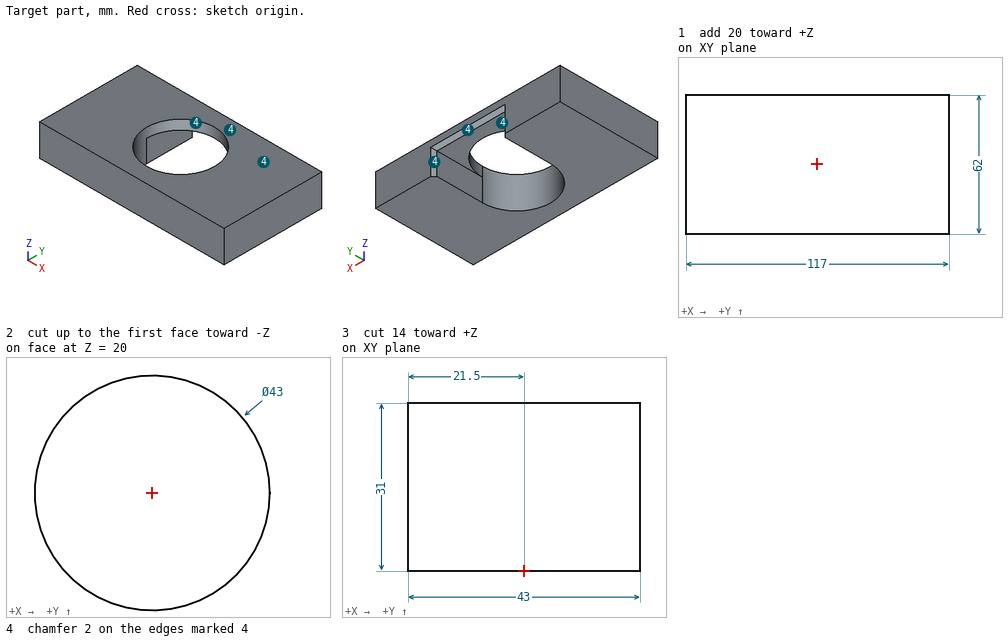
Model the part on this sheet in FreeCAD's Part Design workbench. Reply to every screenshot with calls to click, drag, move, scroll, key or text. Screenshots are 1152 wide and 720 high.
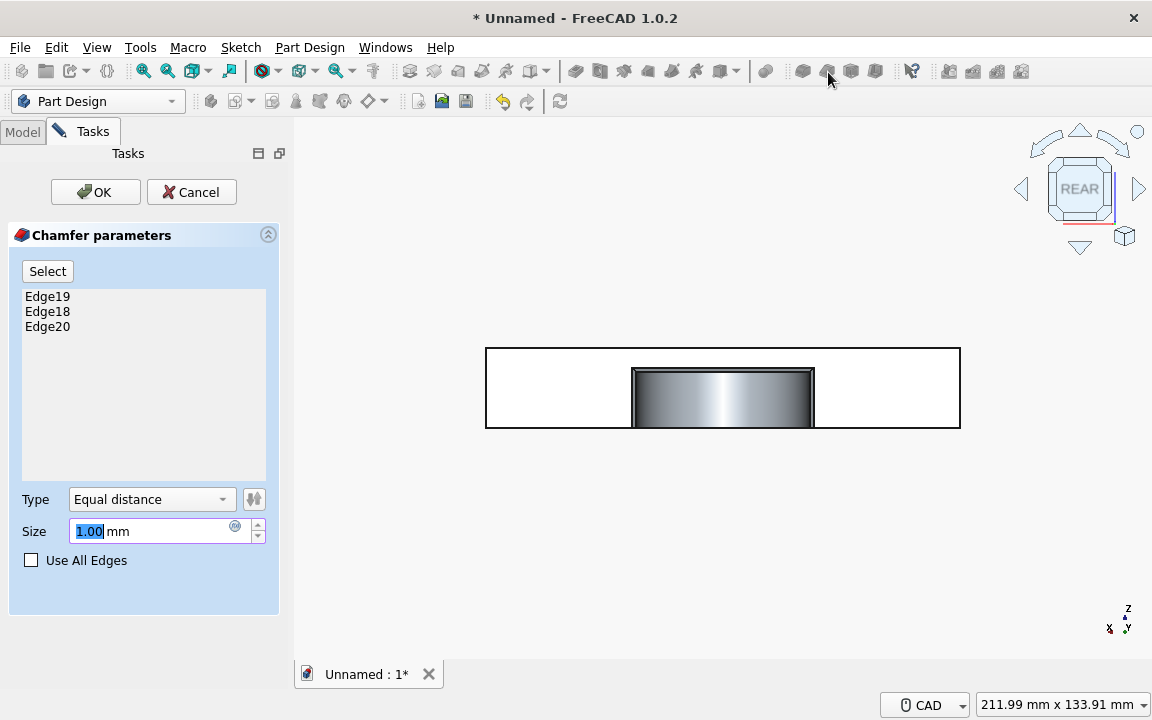
text(2)
key(Tab)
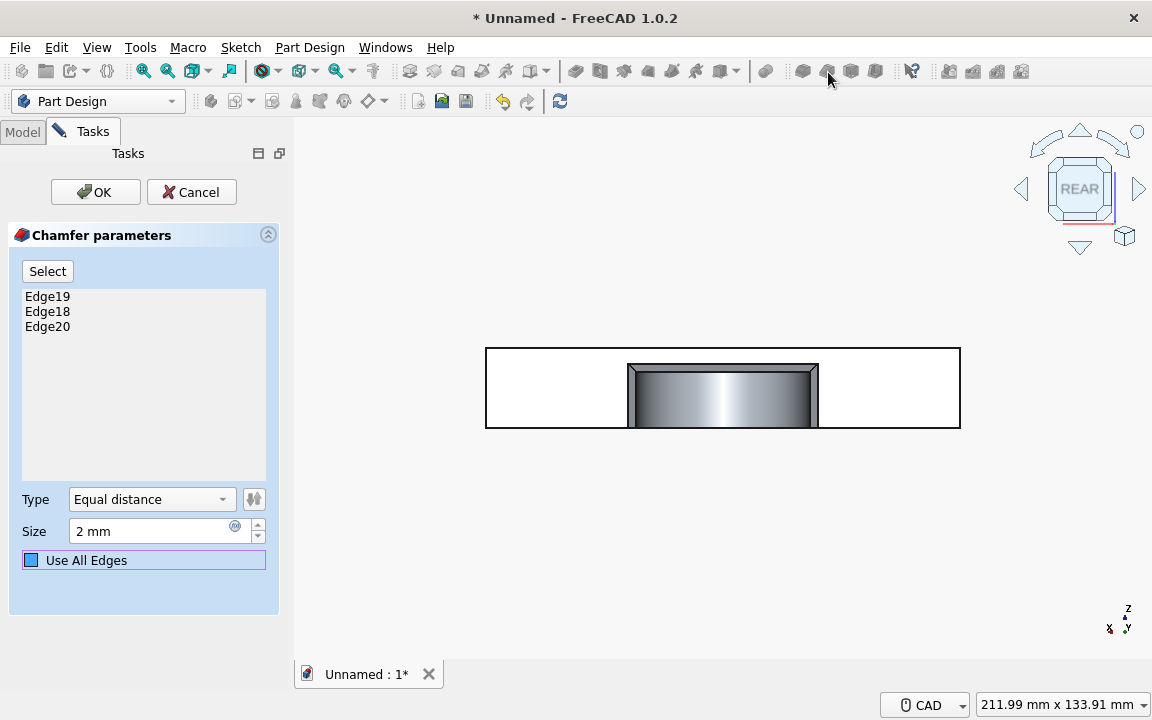
click(96, 192)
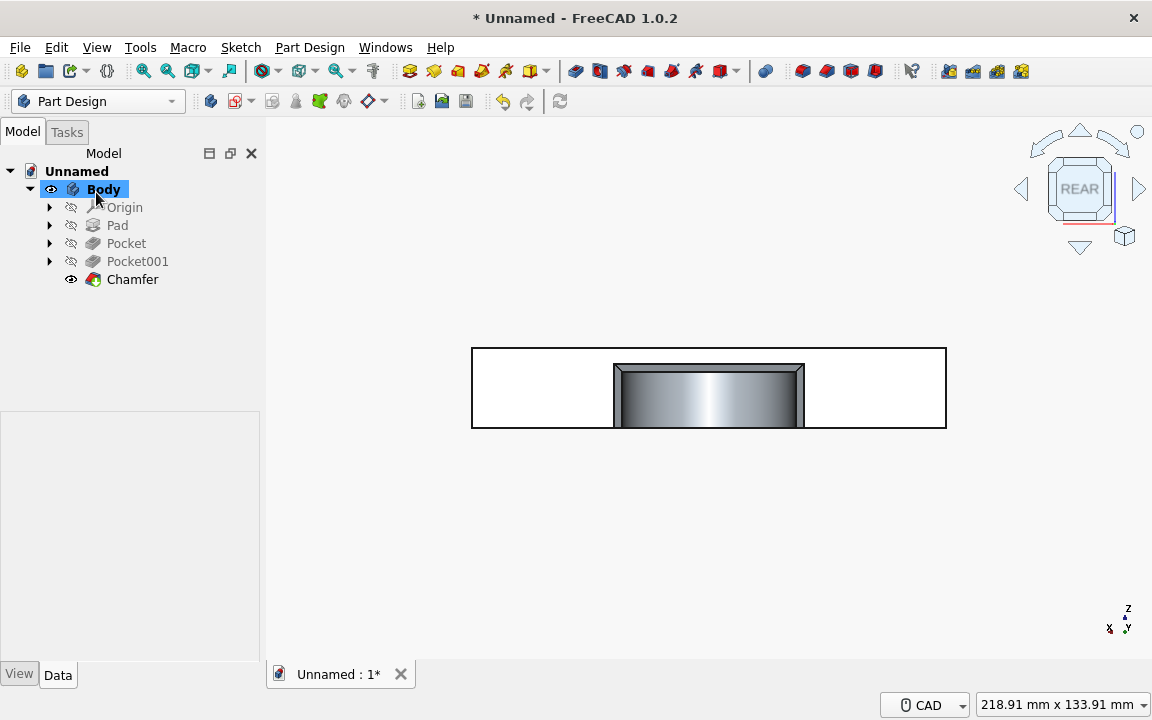
key(0)